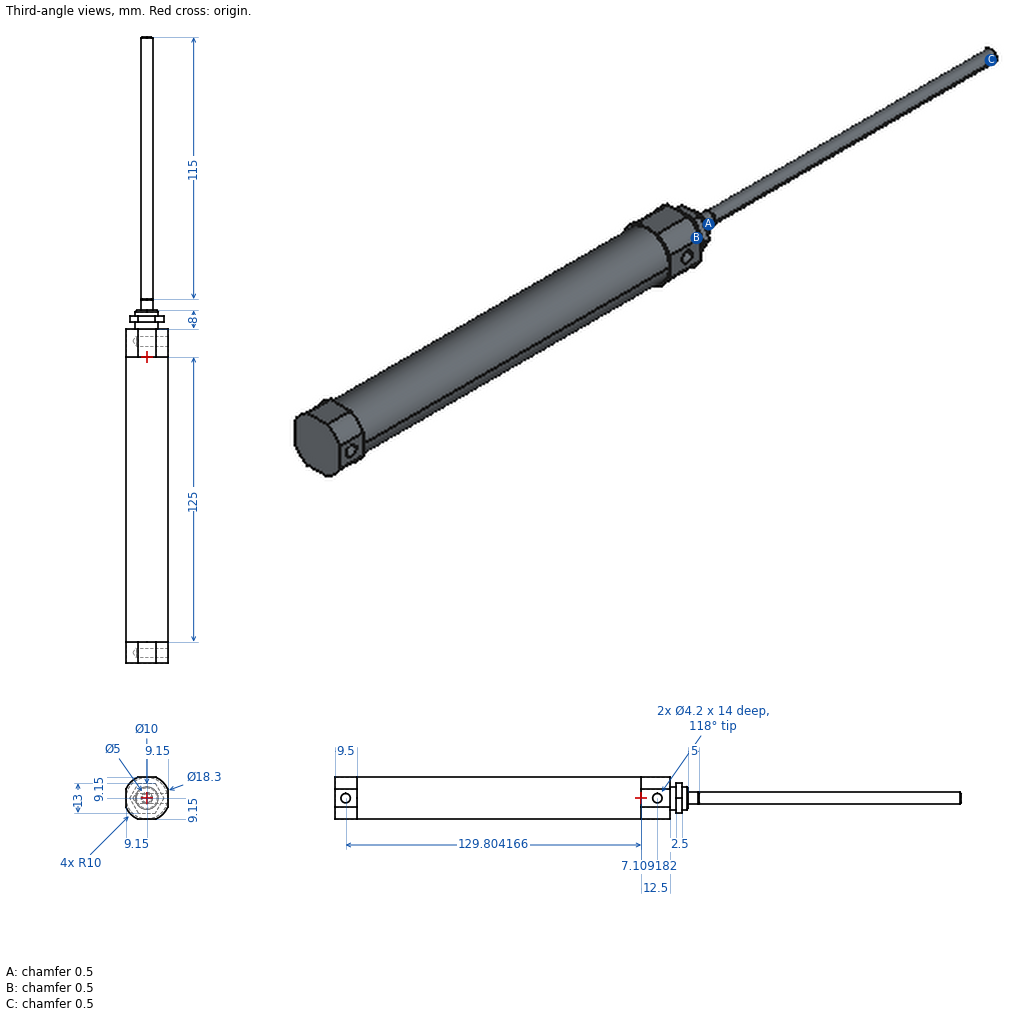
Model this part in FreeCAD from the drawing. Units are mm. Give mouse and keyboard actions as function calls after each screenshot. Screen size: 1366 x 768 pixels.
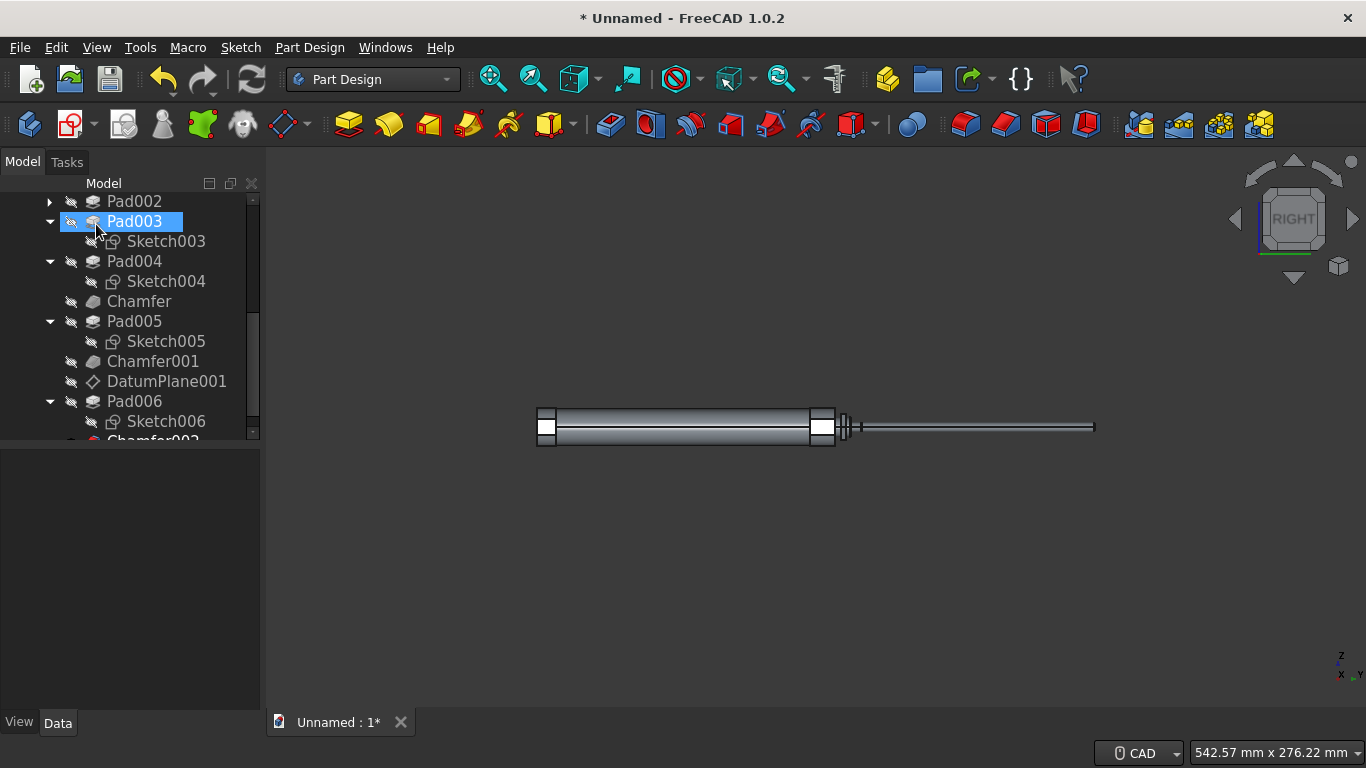
click(826, 426)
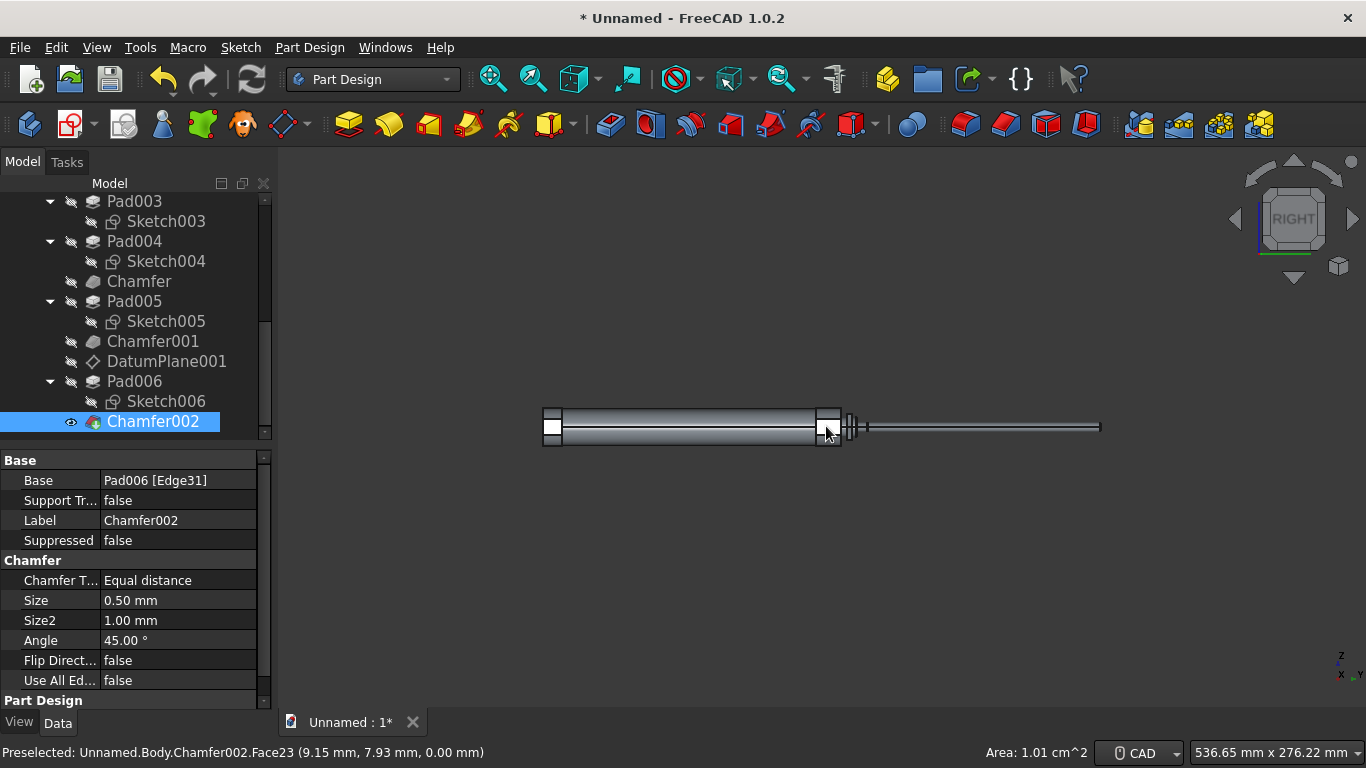
click(70, 124)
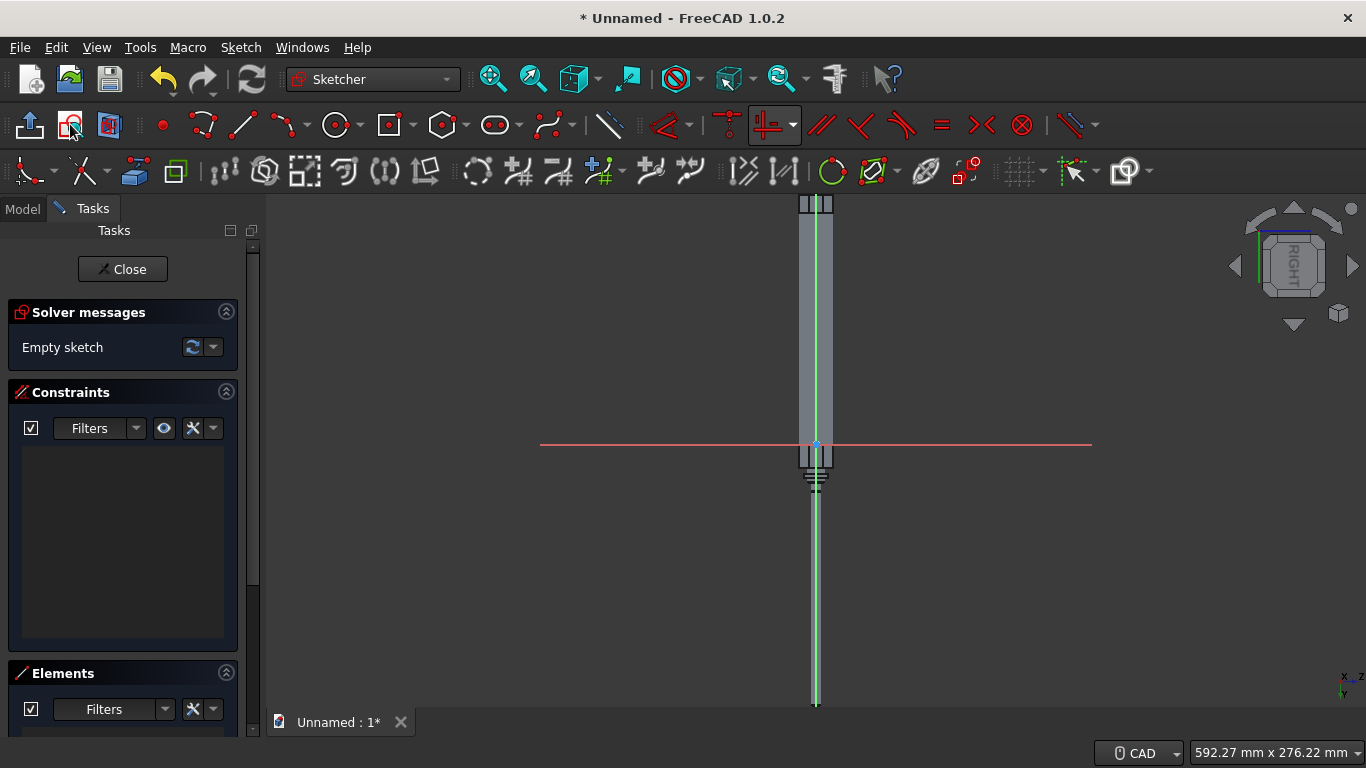
scroll(438, 679, down, 1)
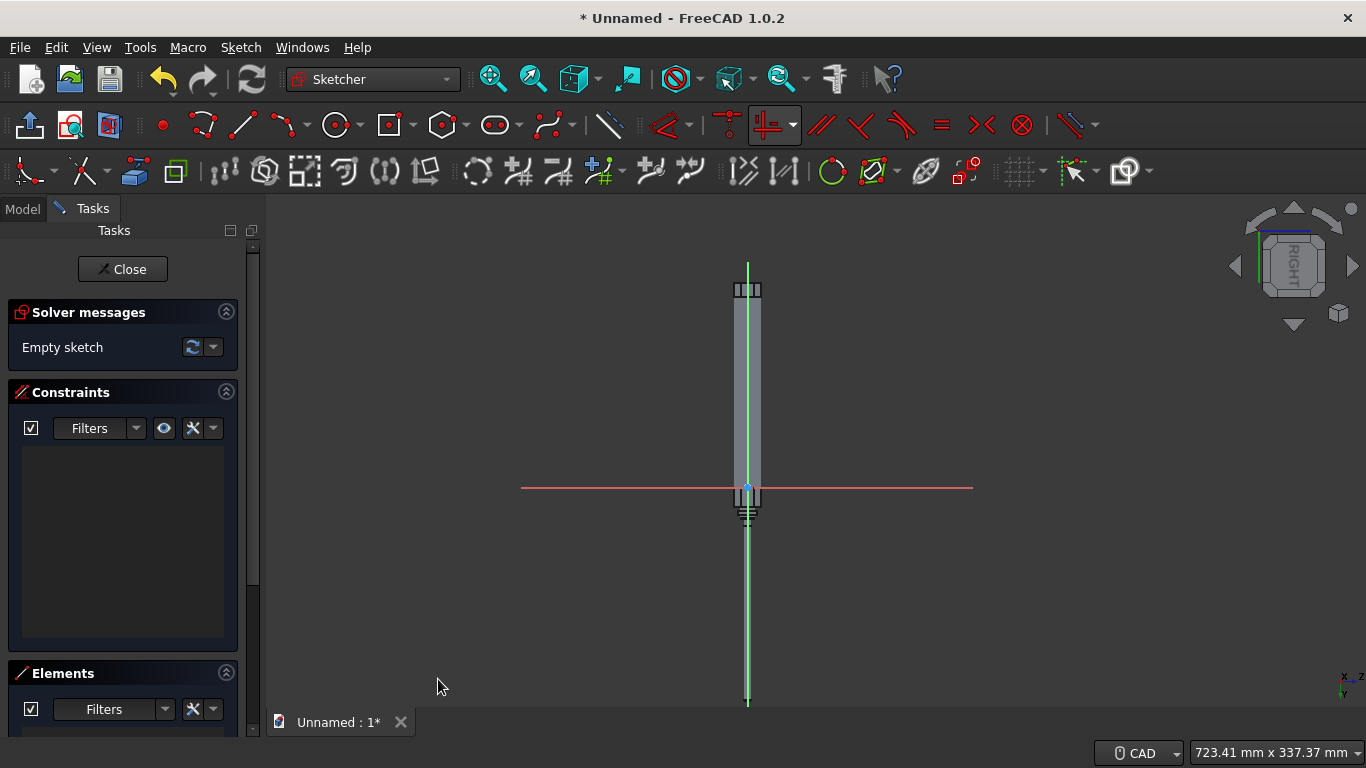
scroll(748, 280, up, 2)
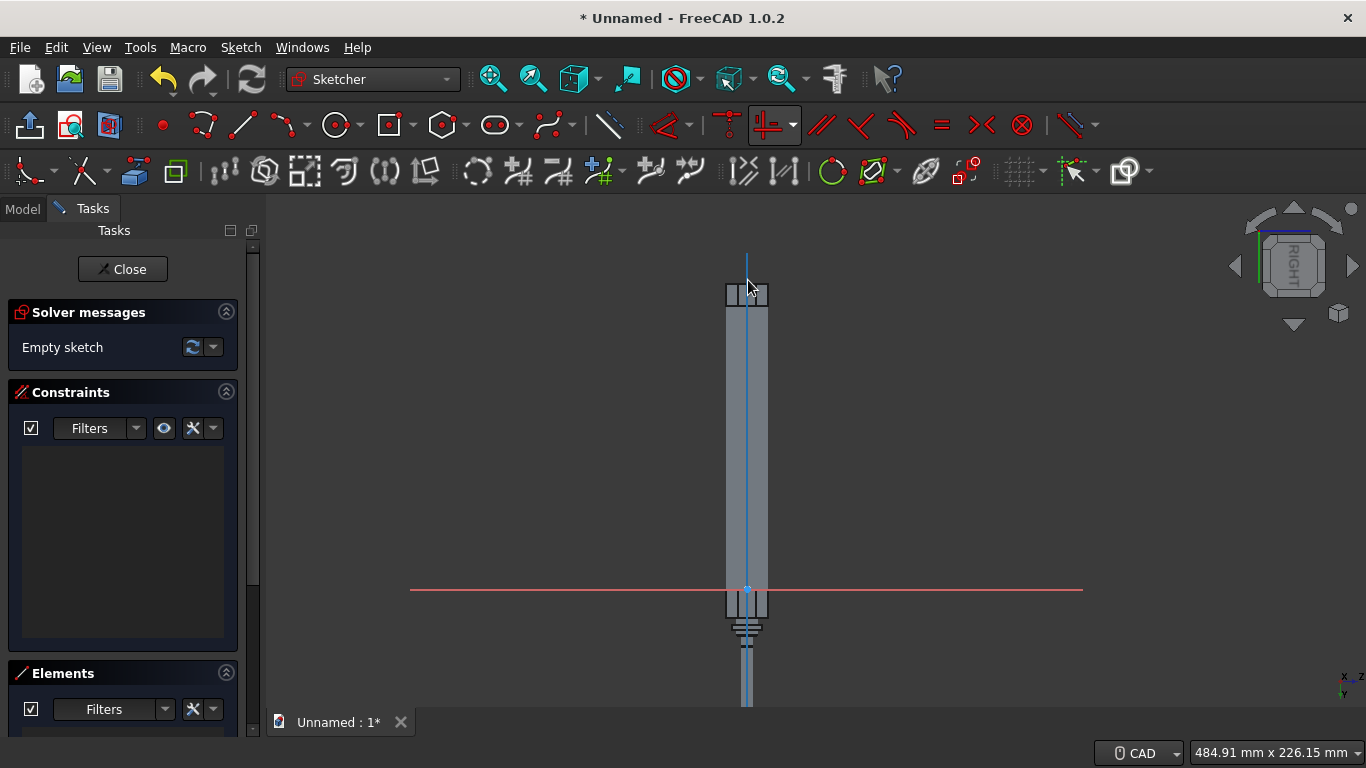
click(336, 126)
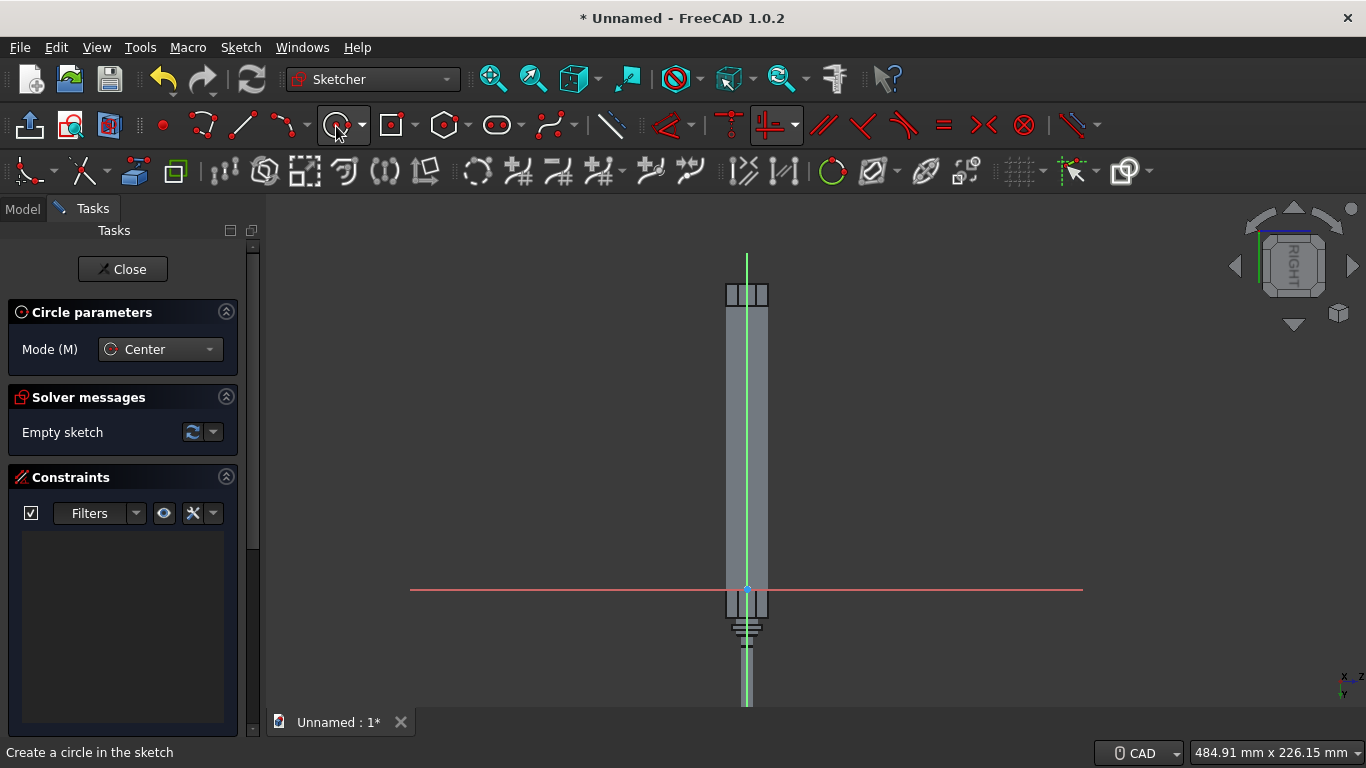
scroll(747, 606, up, 8)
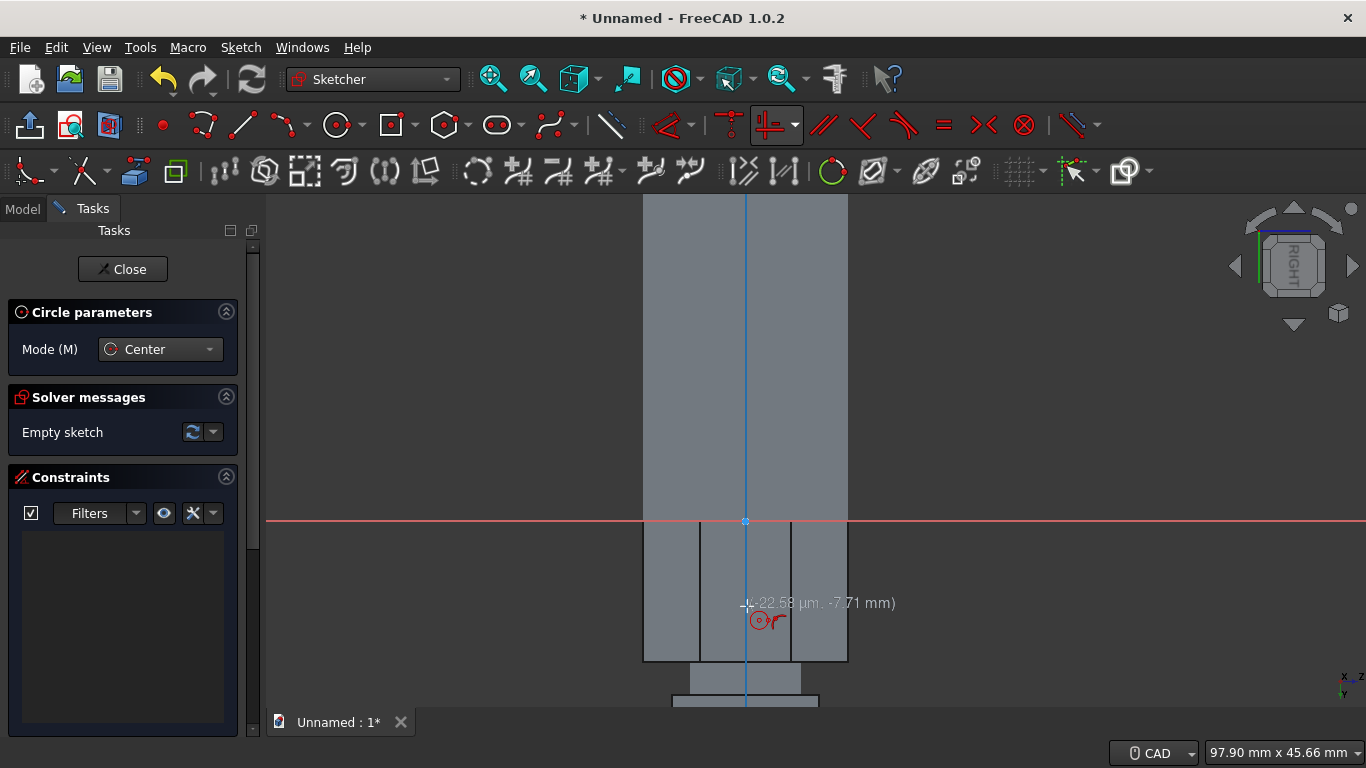
scroll(748, 607, down, 8)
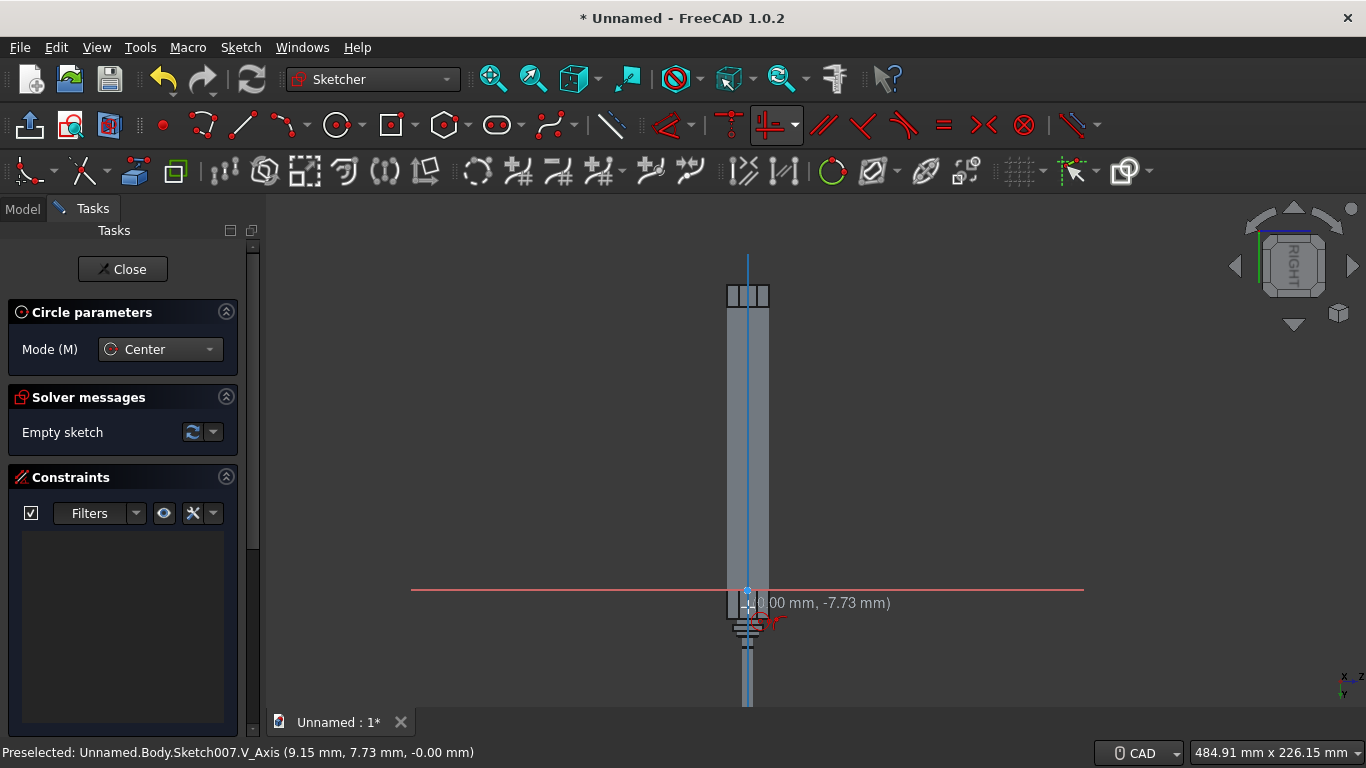
click(748, 606)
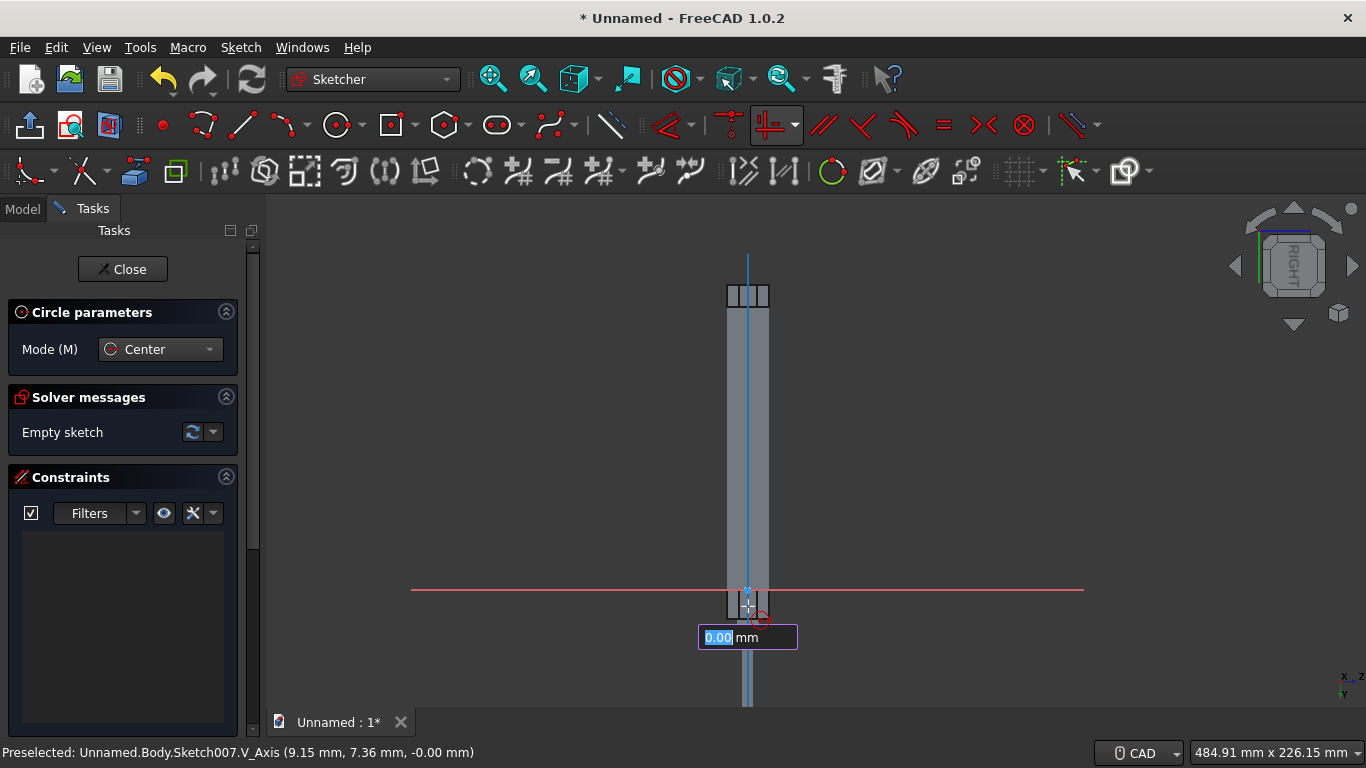
scroll(752, 605, up, 7)